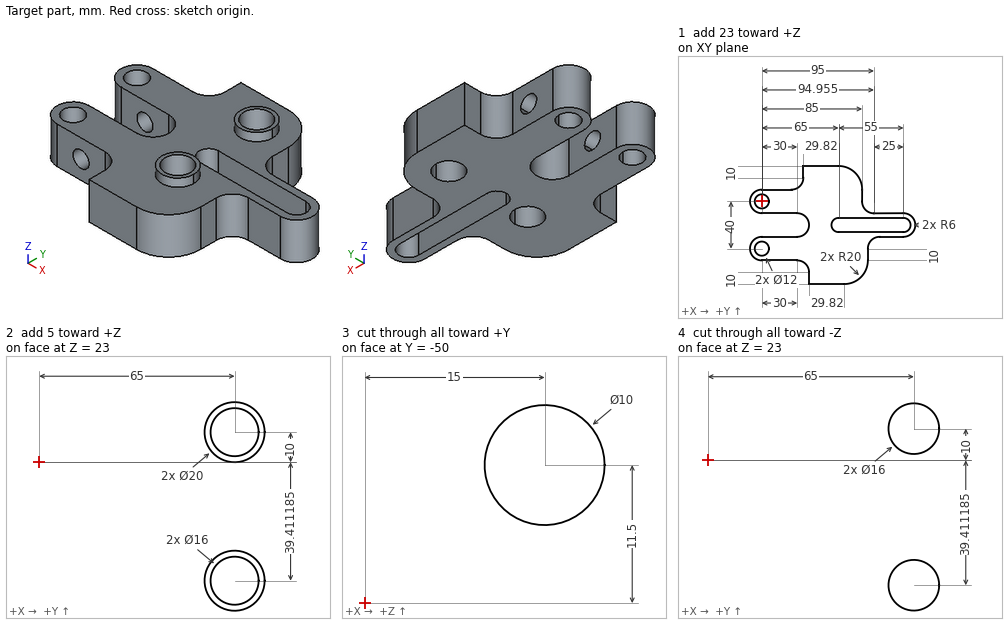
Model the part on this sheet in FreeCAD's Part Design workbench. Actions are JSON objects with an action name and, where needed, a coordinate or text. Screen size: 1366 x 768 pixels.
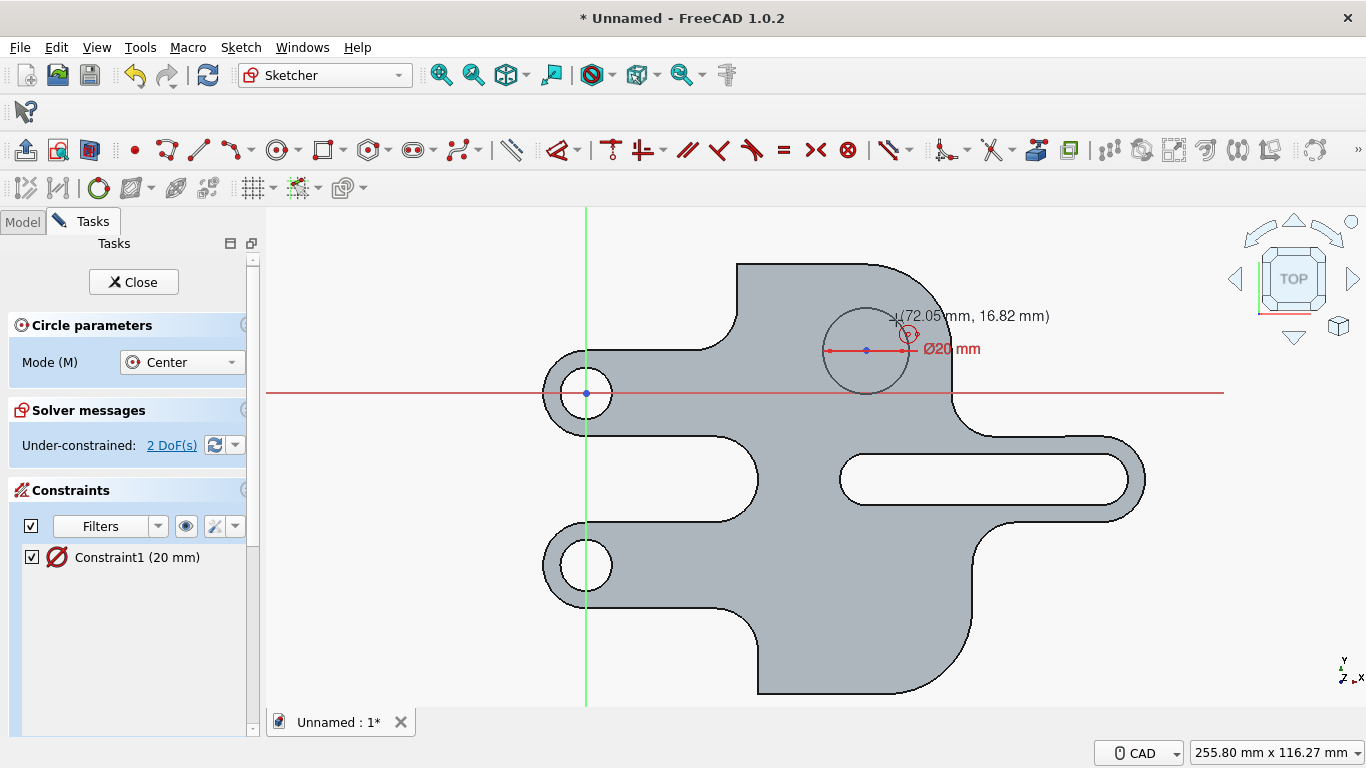
{"action": "left_click", "coordinate": [866, 563]}
{"action": "mouse_move", "coordinate": [896, 532]}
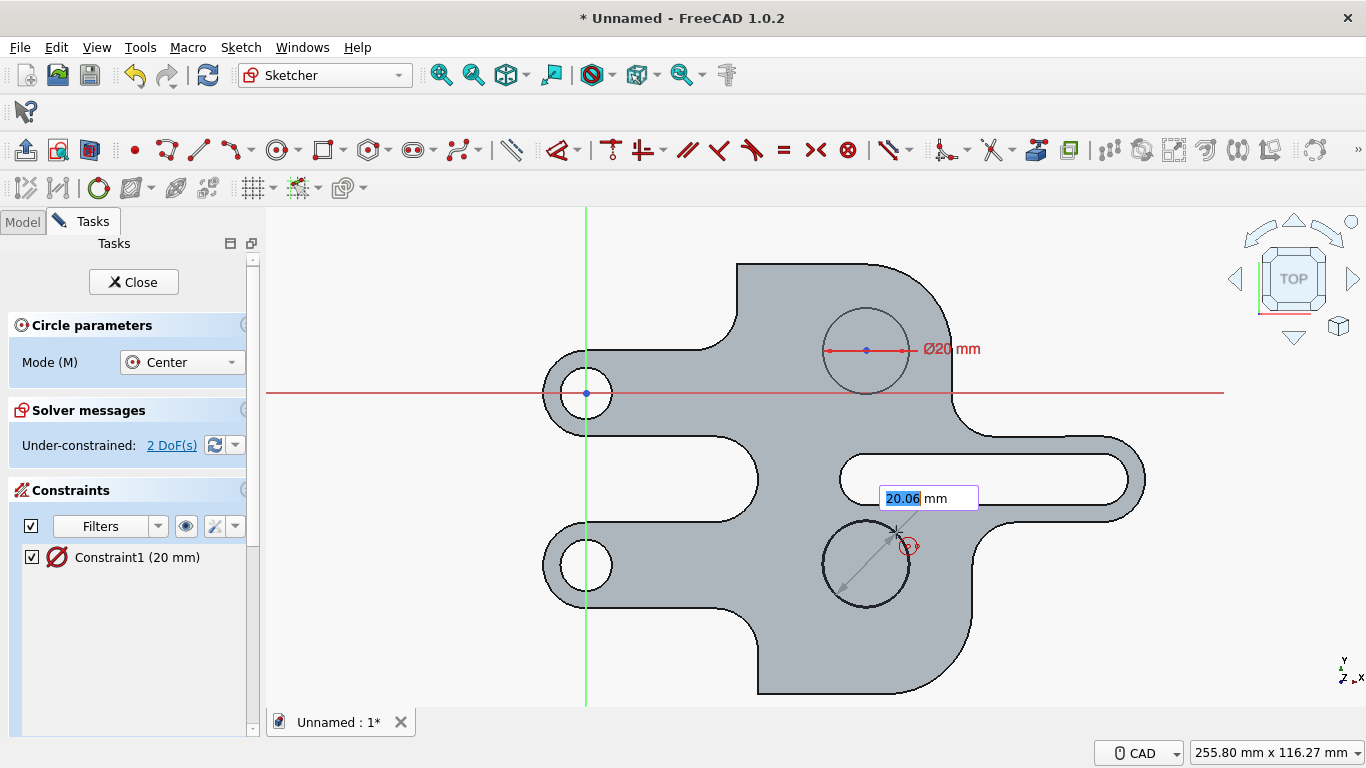
{"action": "type", "text": "20"}
{"action": "key", "text": "Return"}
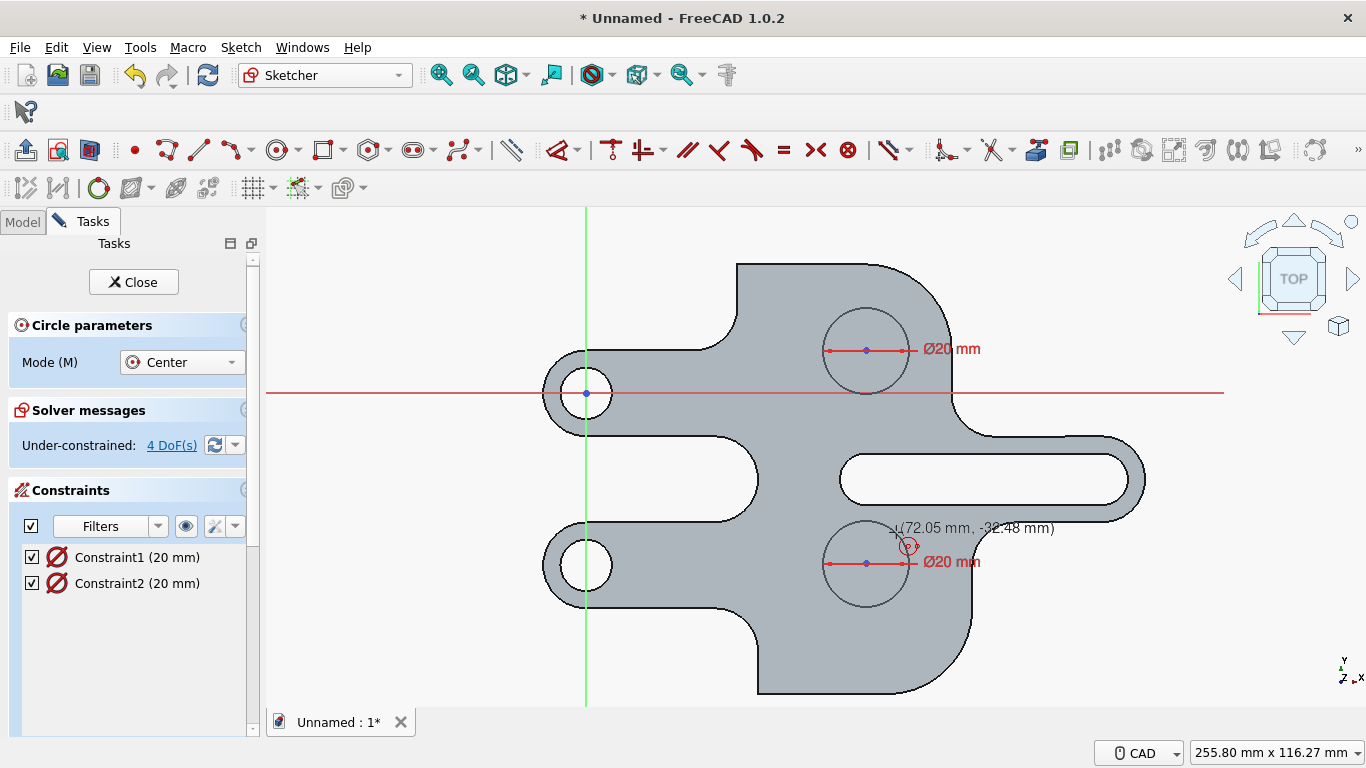
{"action": "left_click", "coordinate": [866, 351]}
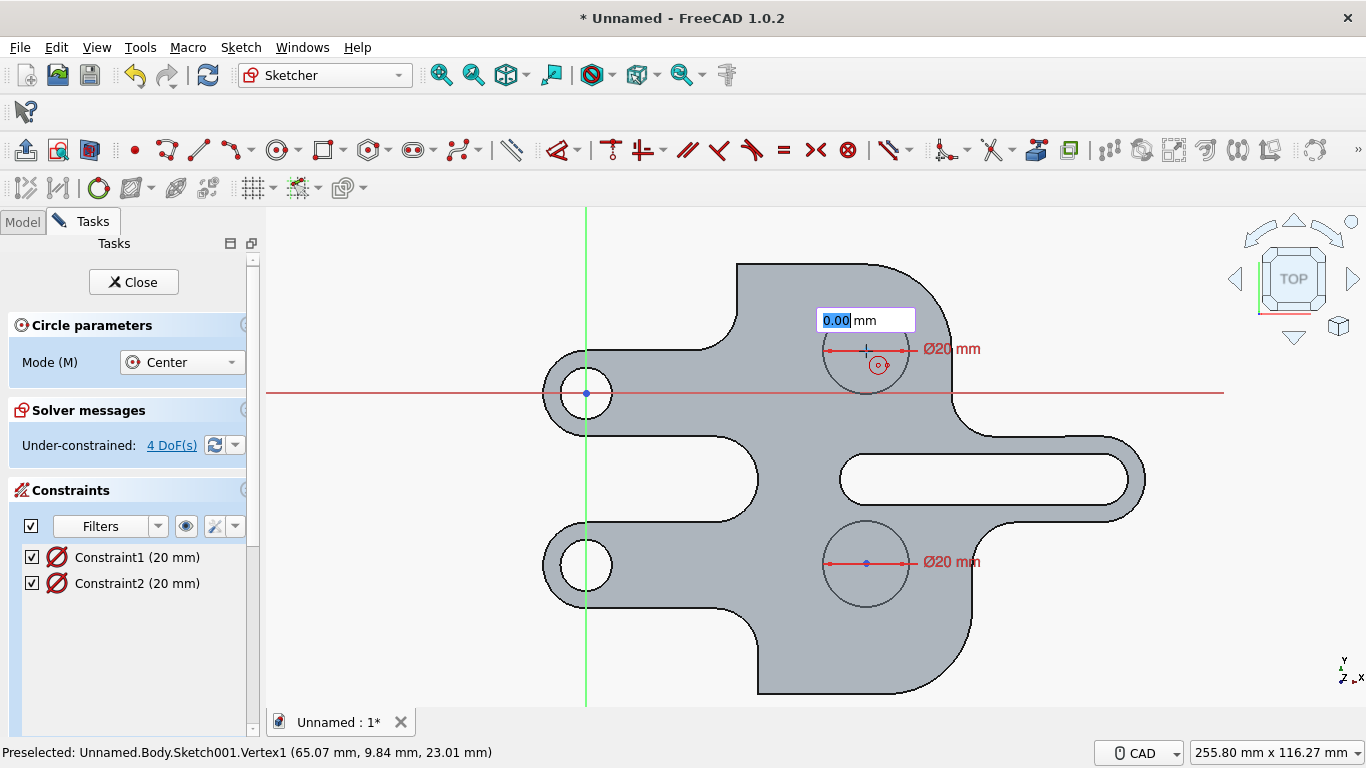
{"action": "scroll", "coordinate": [833, 339], "scroll_direction": "up", "scroll_amount": 4}
{"action": "mouse_move", "coordinate": [833, 338]}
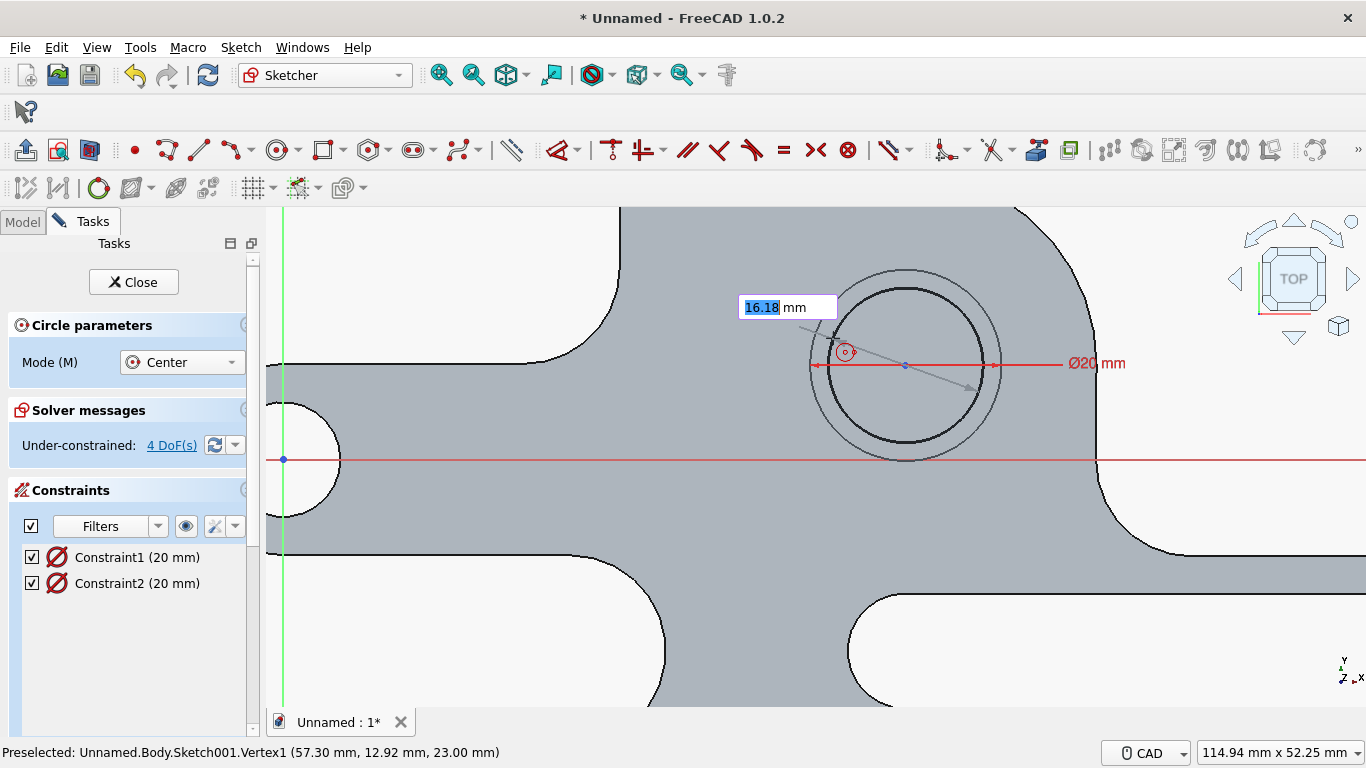
{"action": "type", "text": "16"}
{"action": "key", "text": "Return"}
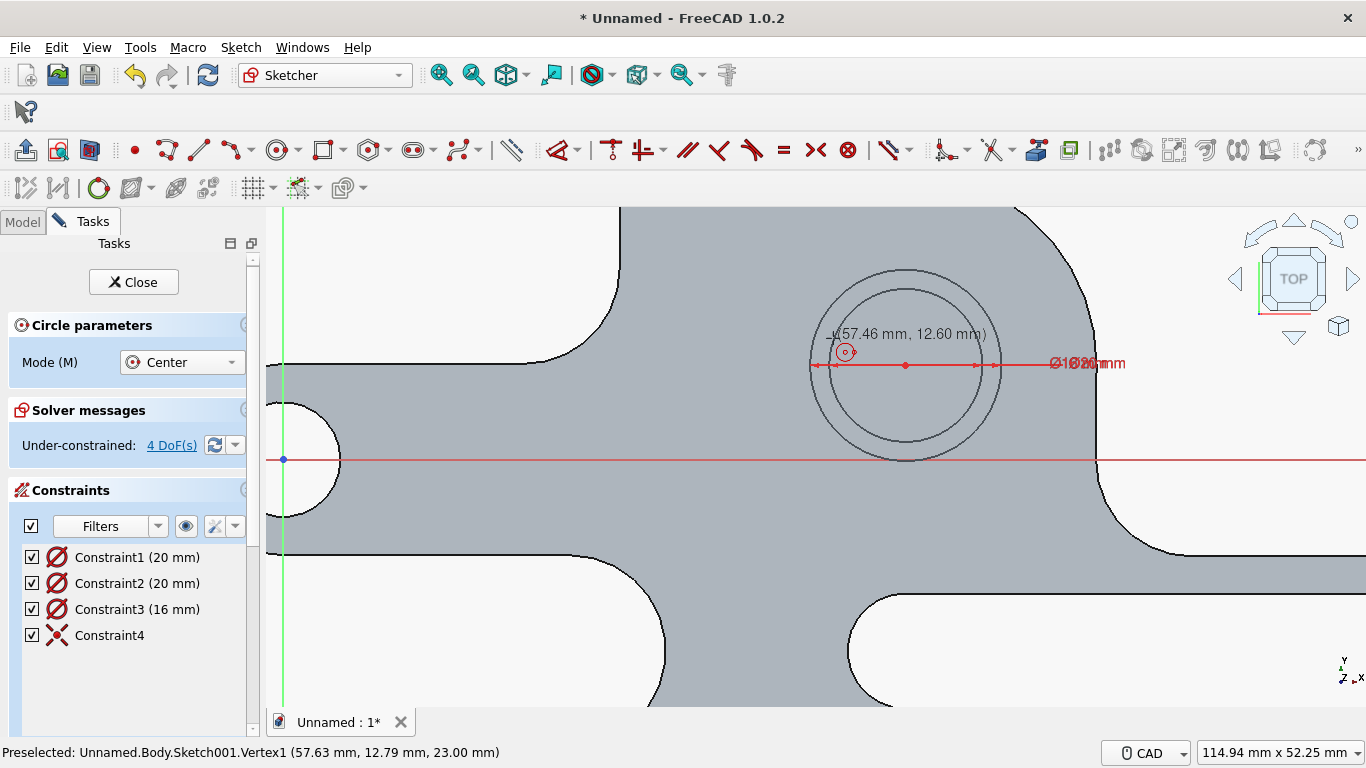
{"action": "scroll", "coordinate": [834, 340], "scroll_direction": "down", "scroll_amount": 4}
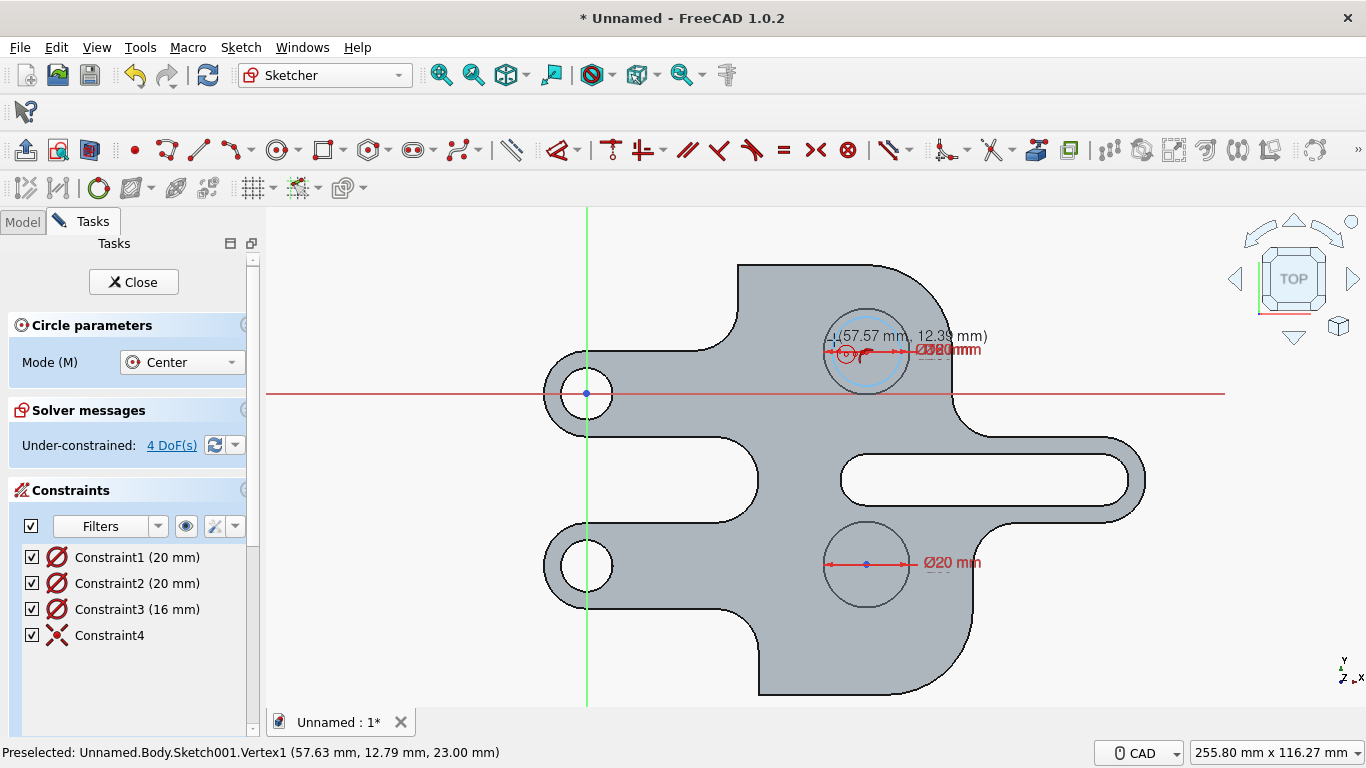
{"action": "left_click", "coordinate": [867, 565]}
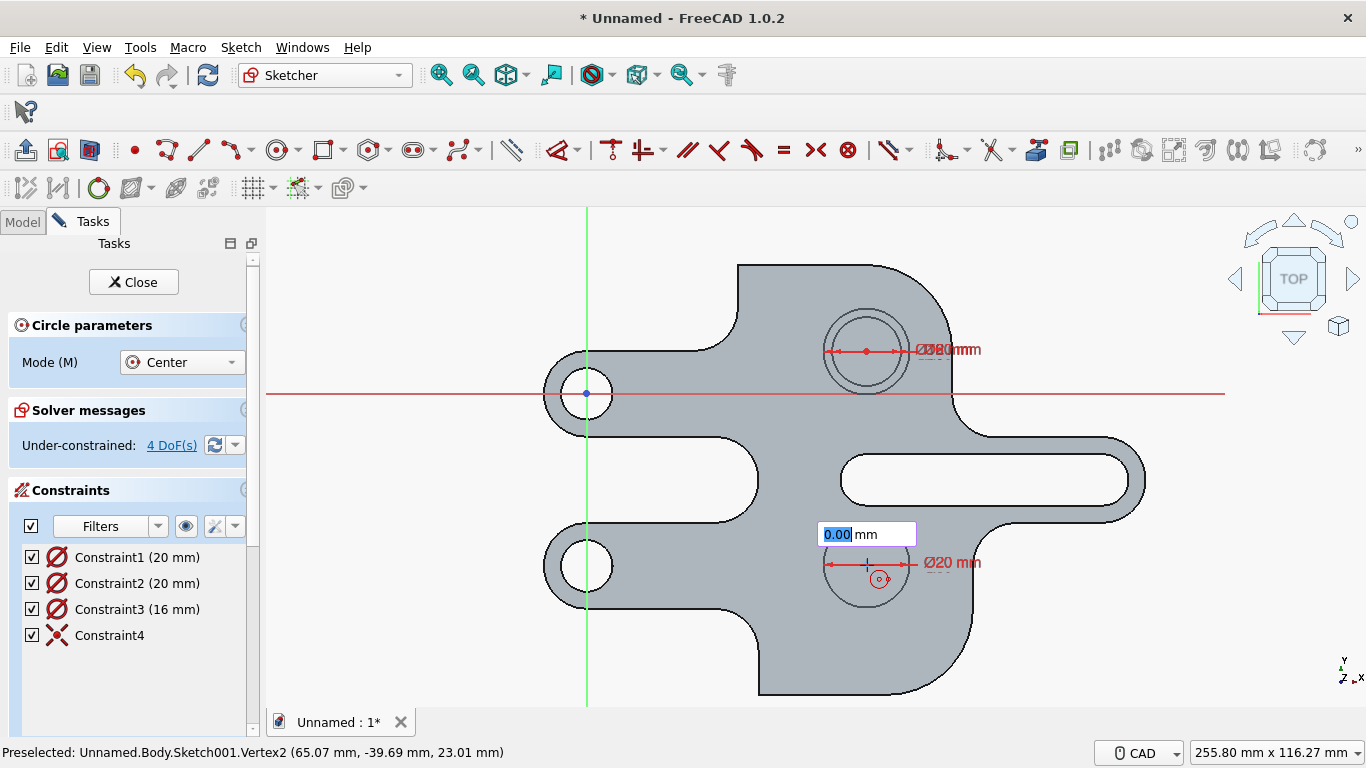
{"action": "scroll", "coordinate": [834, 552], "scroll_direction": "up", "scroll_amount": 4}
{"action": "mouse_move", "coordinate": [833, 550]}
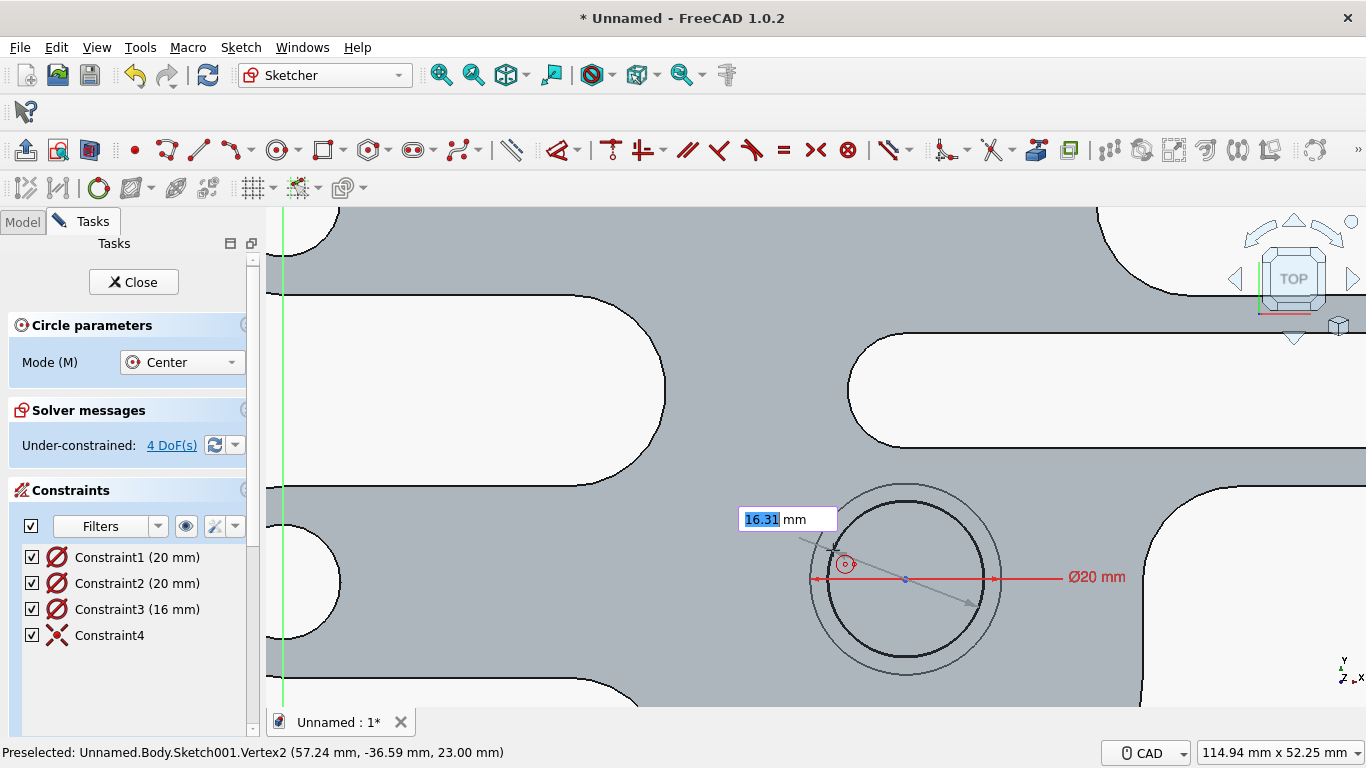
{"action": "type", "text": "16"}
{"action": "key", "text": "Return"}
{"action": "key", "text": "Escape"}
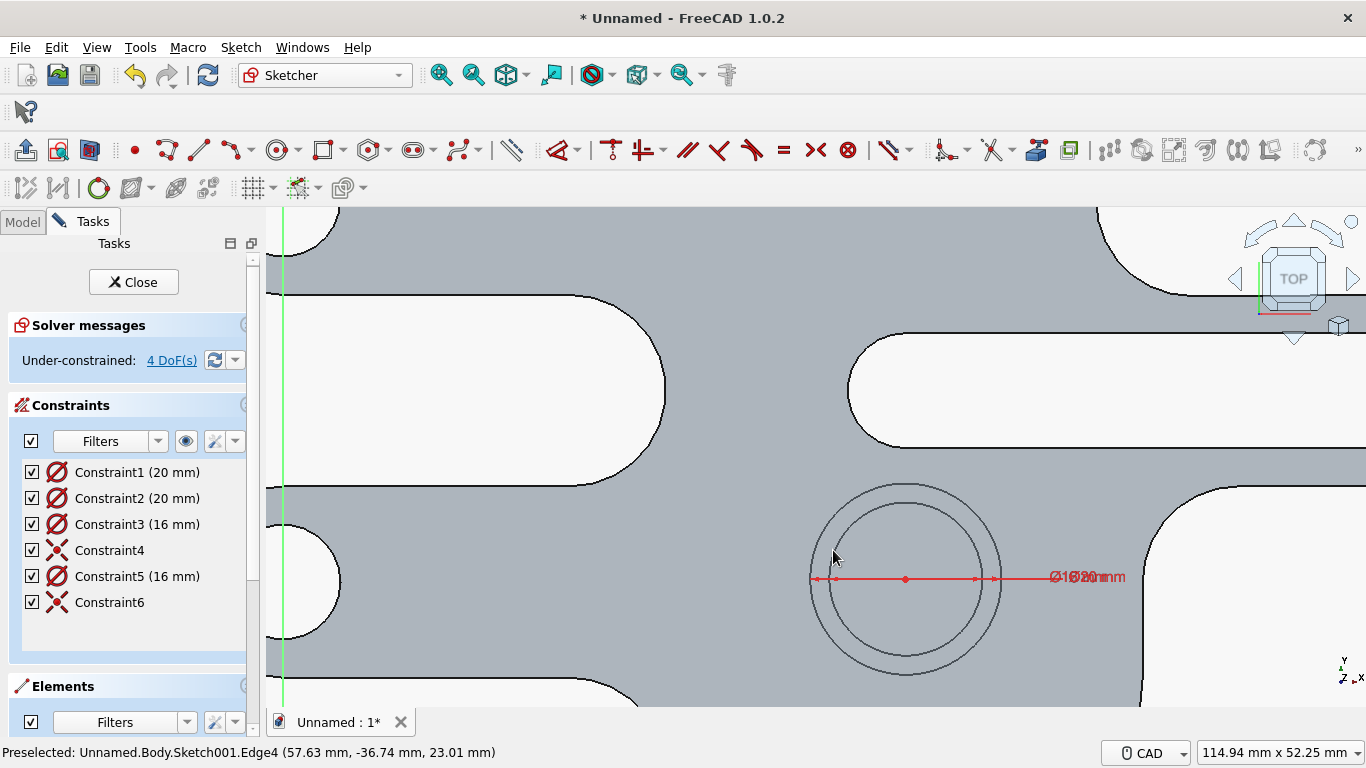
{"action": "scroll", "coordinate": [834, 552], "scroll_direction": "down", "scroll_amount": 4}